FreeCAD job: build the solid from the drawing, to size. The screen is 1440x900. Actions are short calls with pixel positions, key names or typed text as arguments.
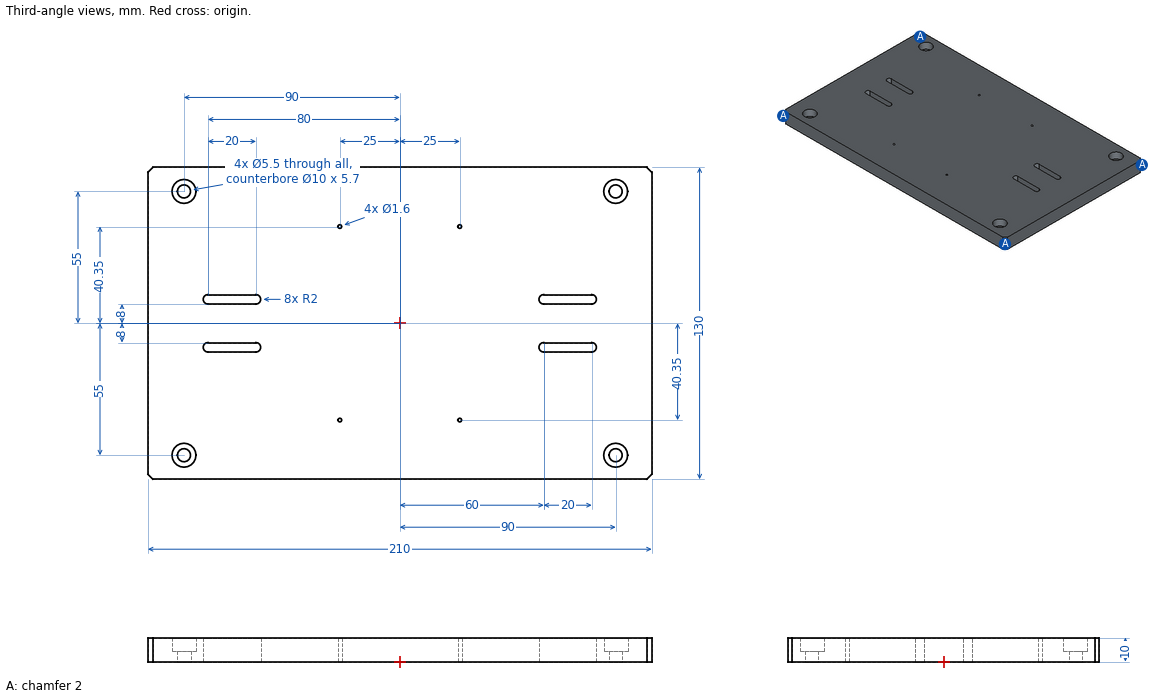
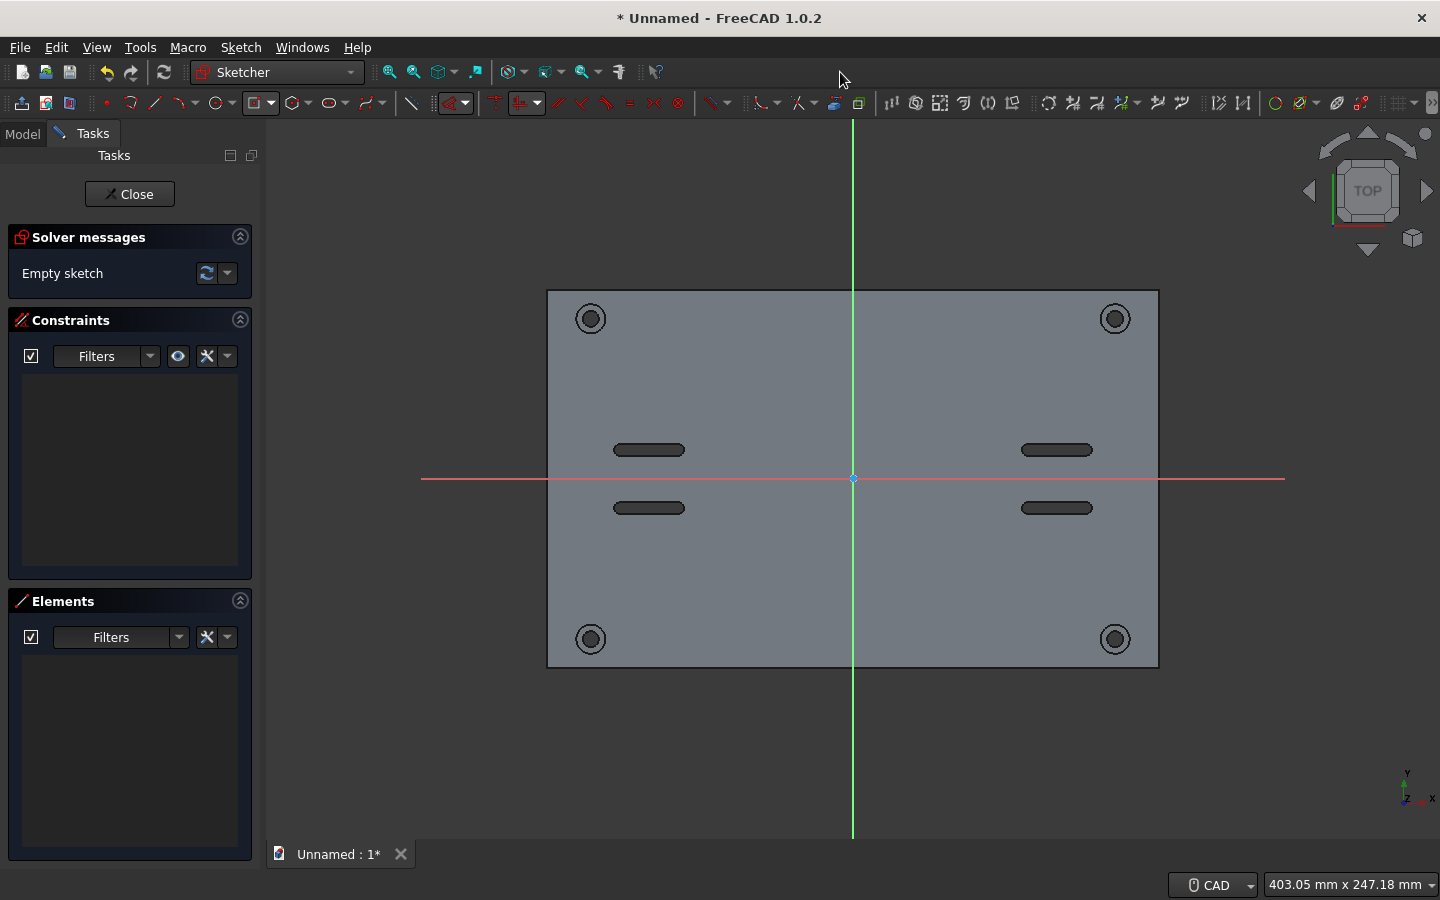
scroll(936, 479, up, 3)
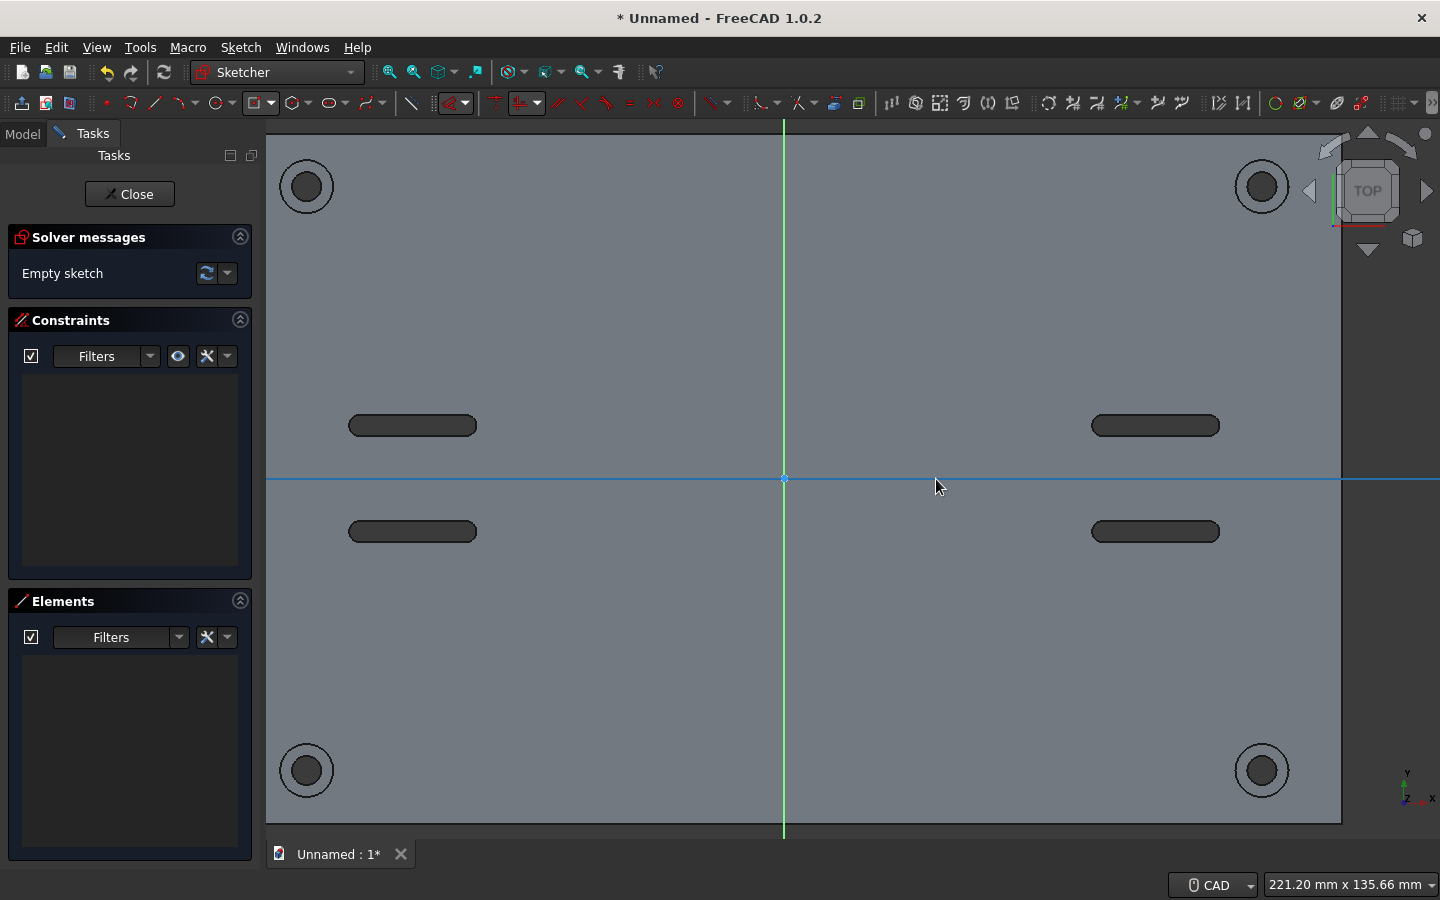
click(216, 104)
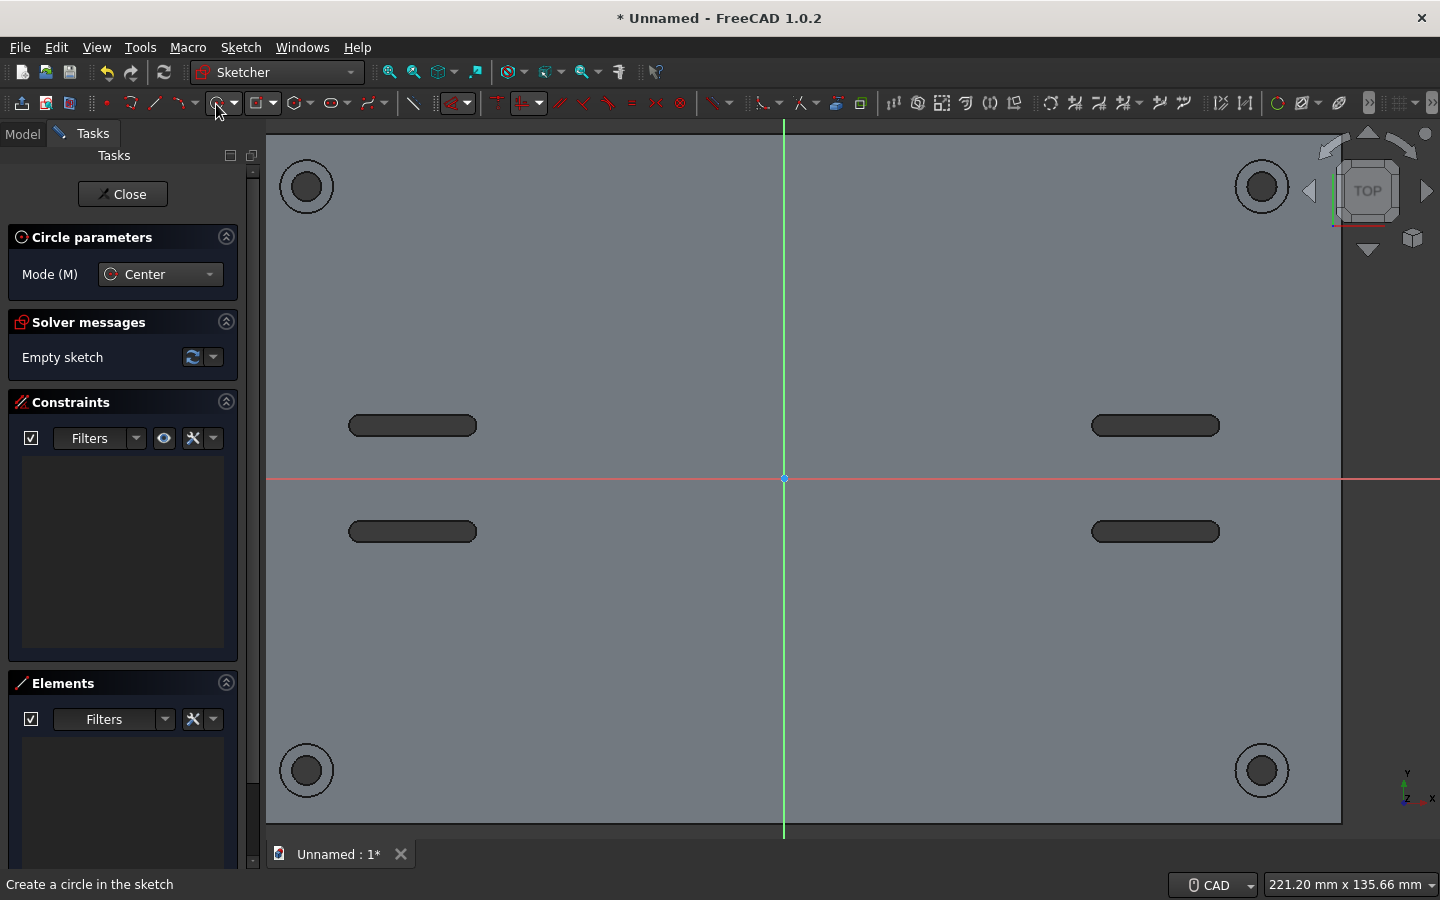
scroll(652, 264, up, 9)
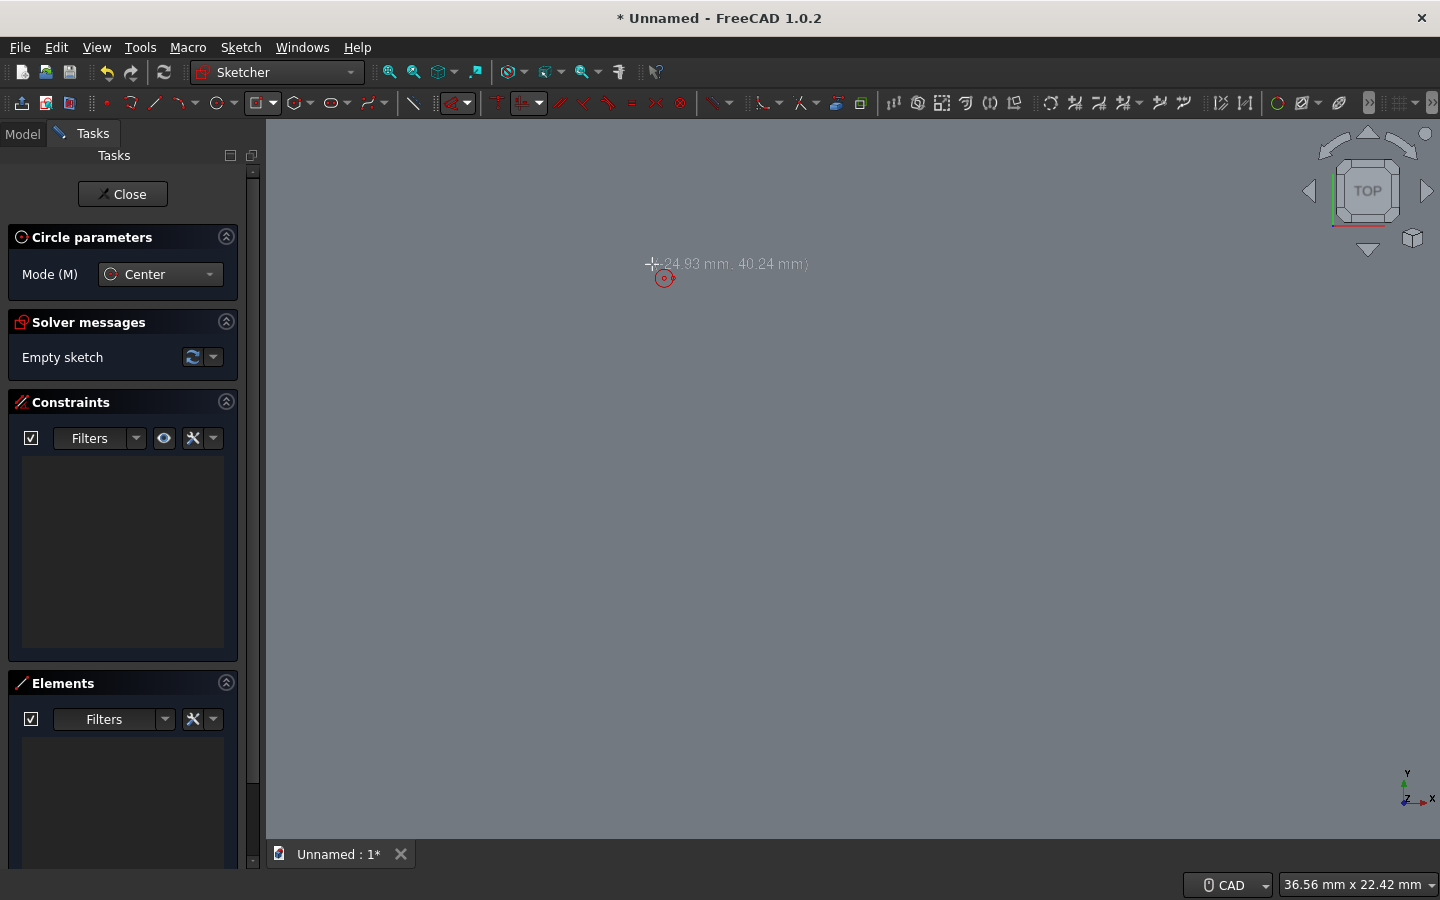
scroll(653, 265, down, 9)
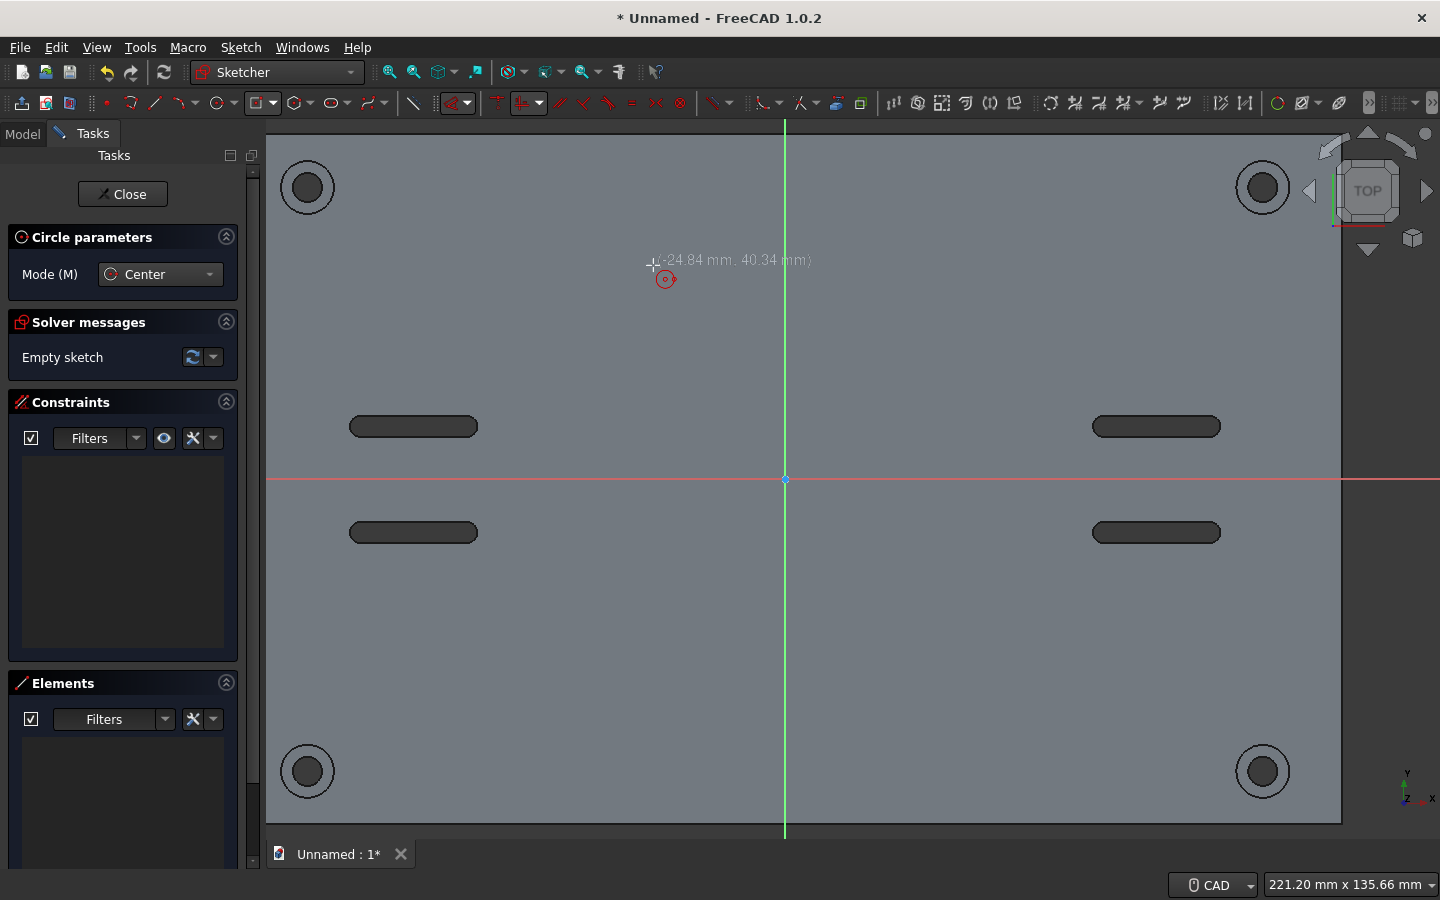
click(652, 265)
move(655, 262)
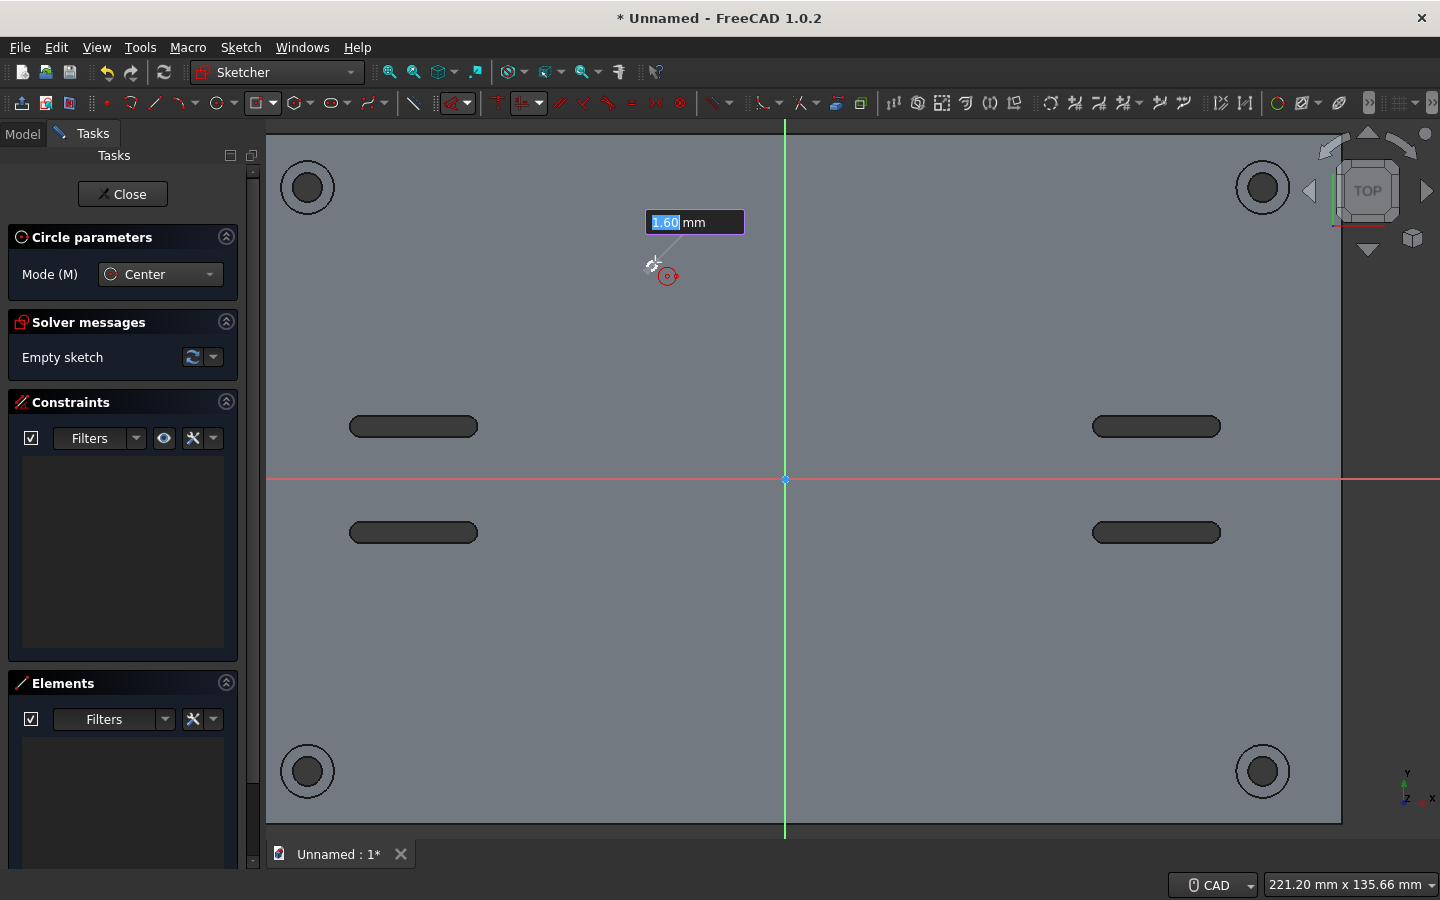
text(1.6)
key(Return)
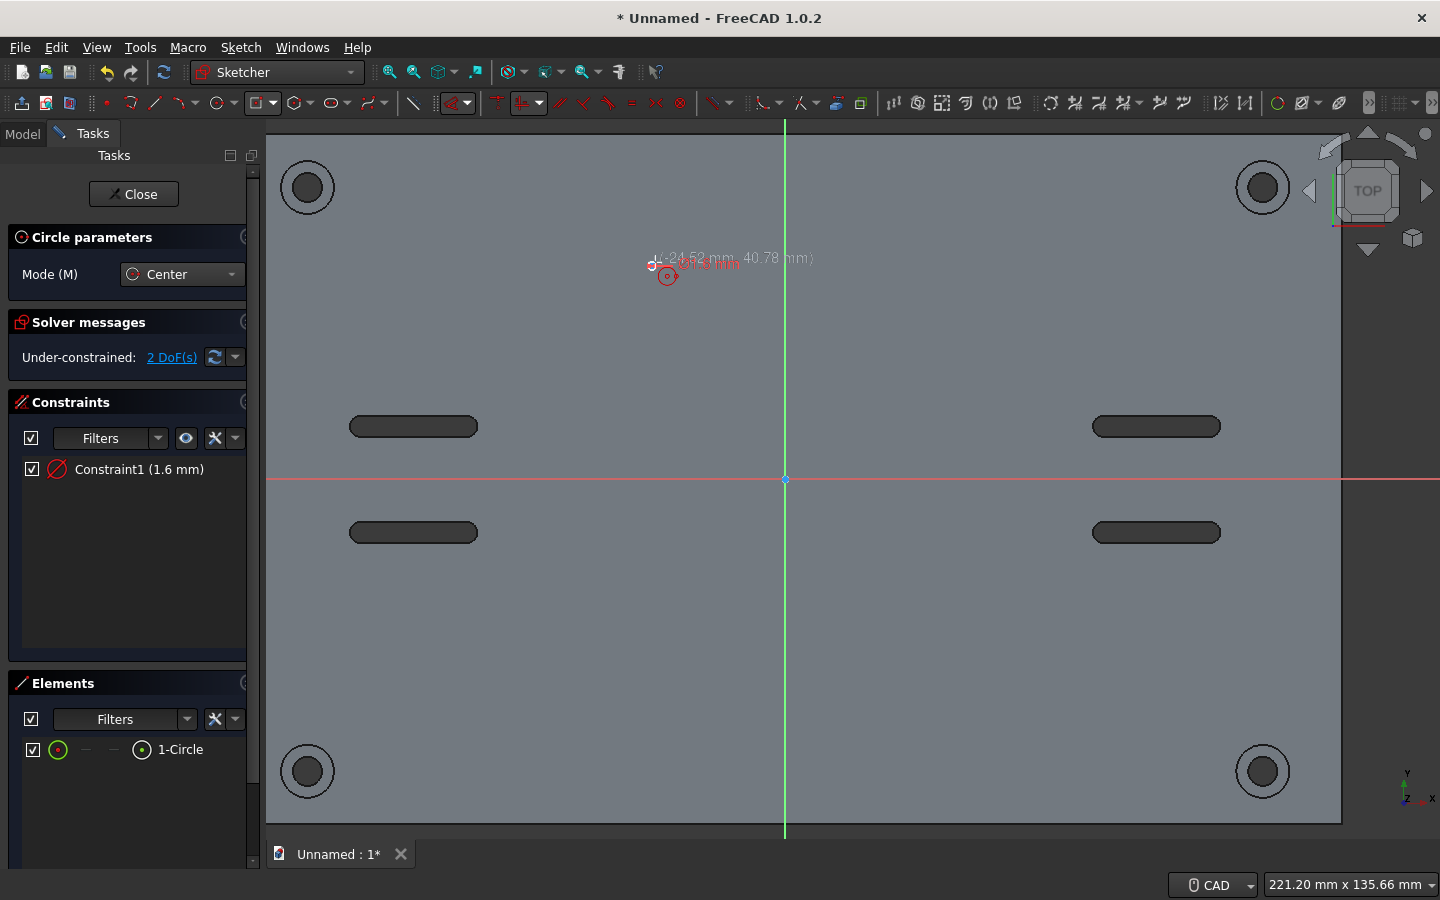
scroll(918, 265, up, 9)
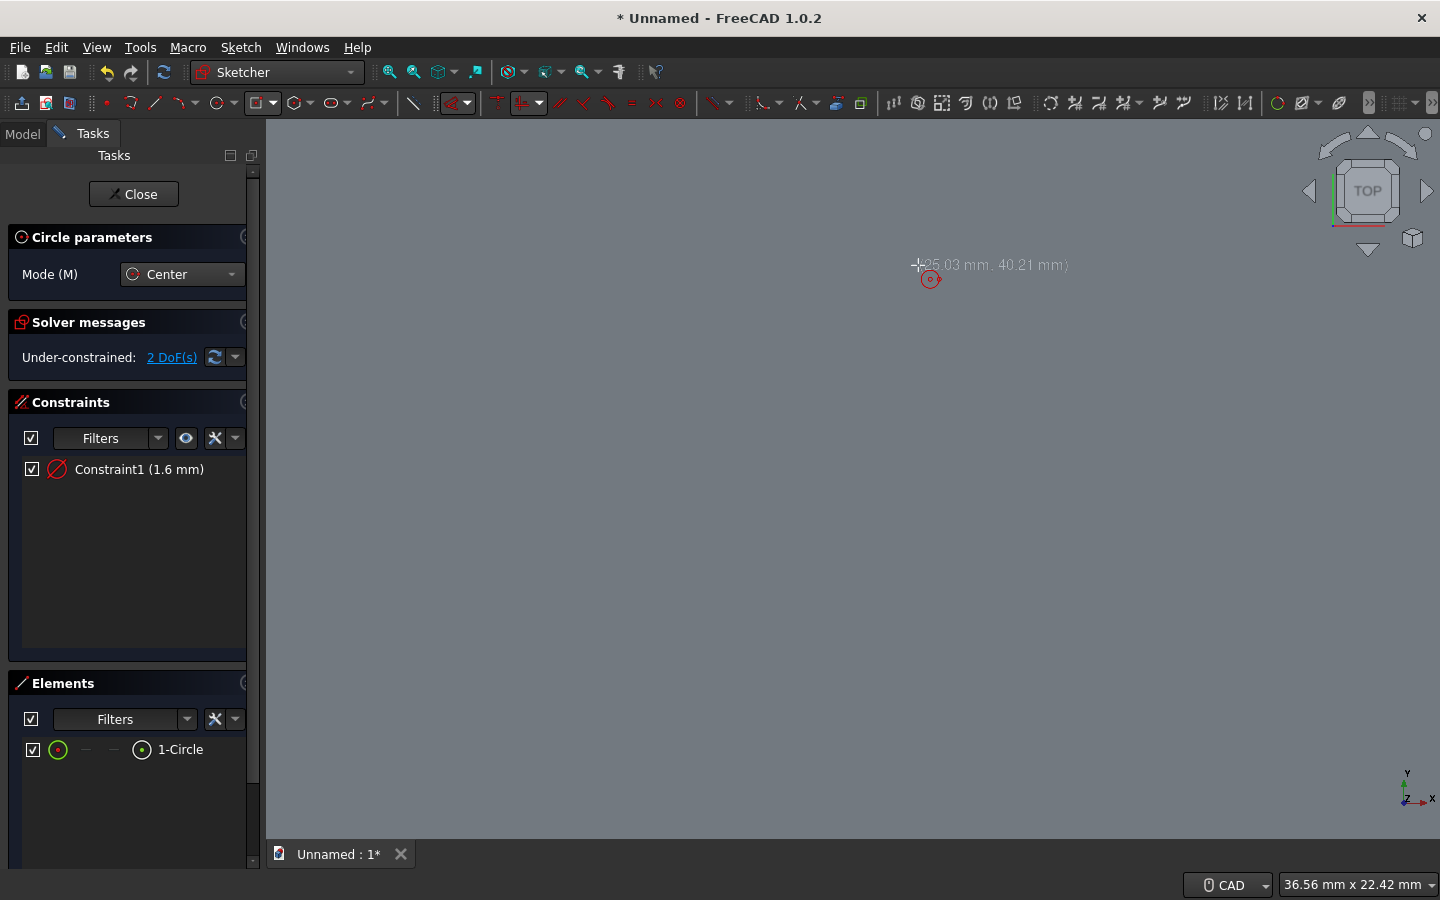
scroll(918, 265, down, 9)